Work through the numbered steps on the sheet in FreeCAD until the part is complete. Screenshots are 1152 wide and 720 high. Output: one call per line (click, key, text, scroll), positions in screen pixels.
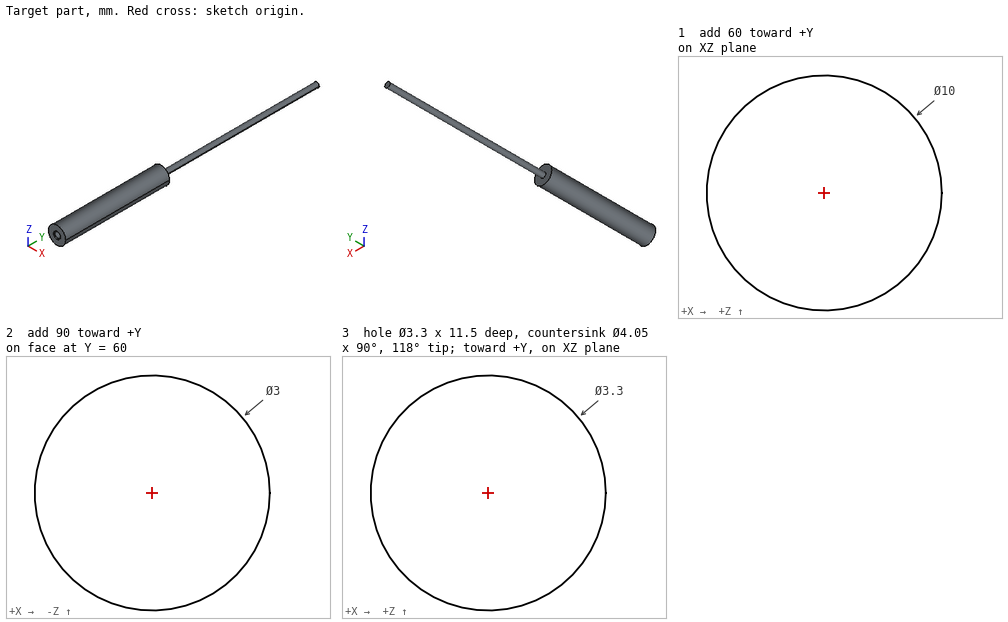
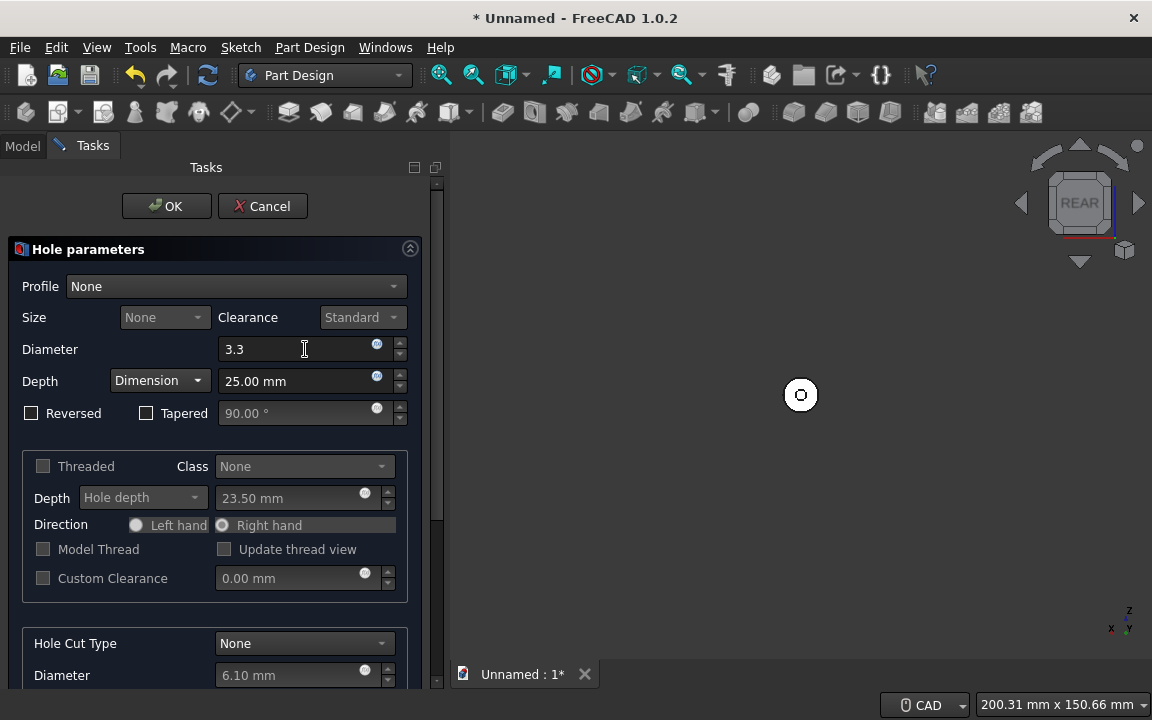
triple_click(305, 381)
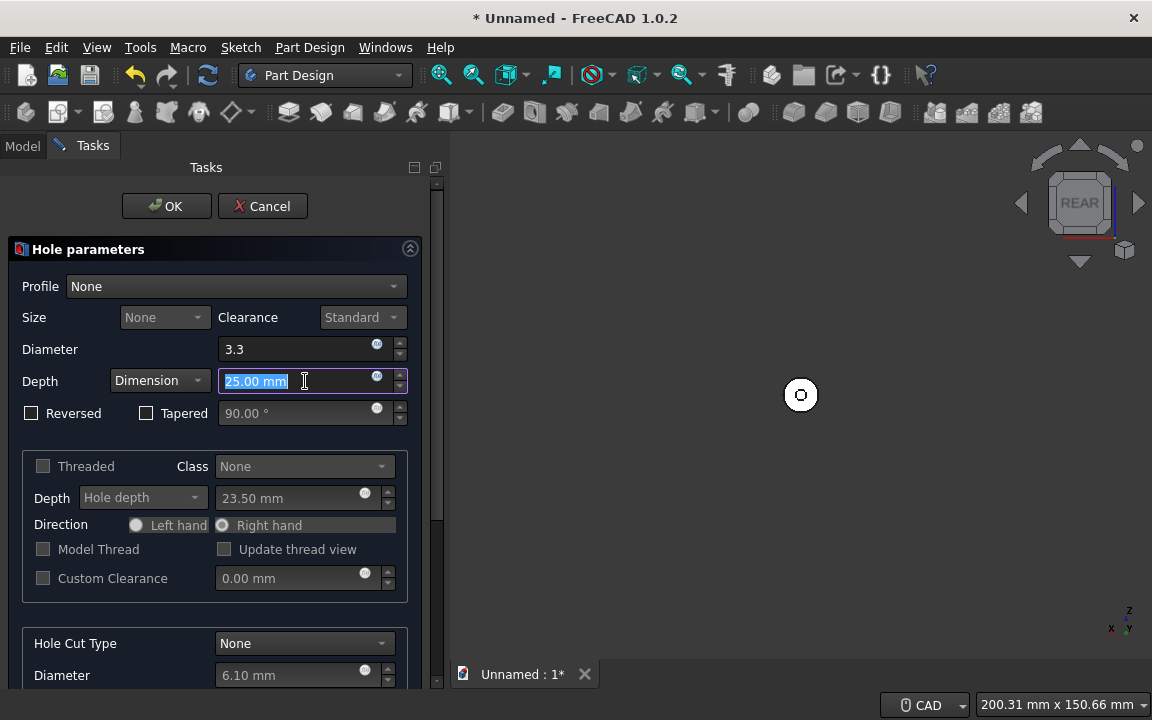
text(11.5)
key(Tab)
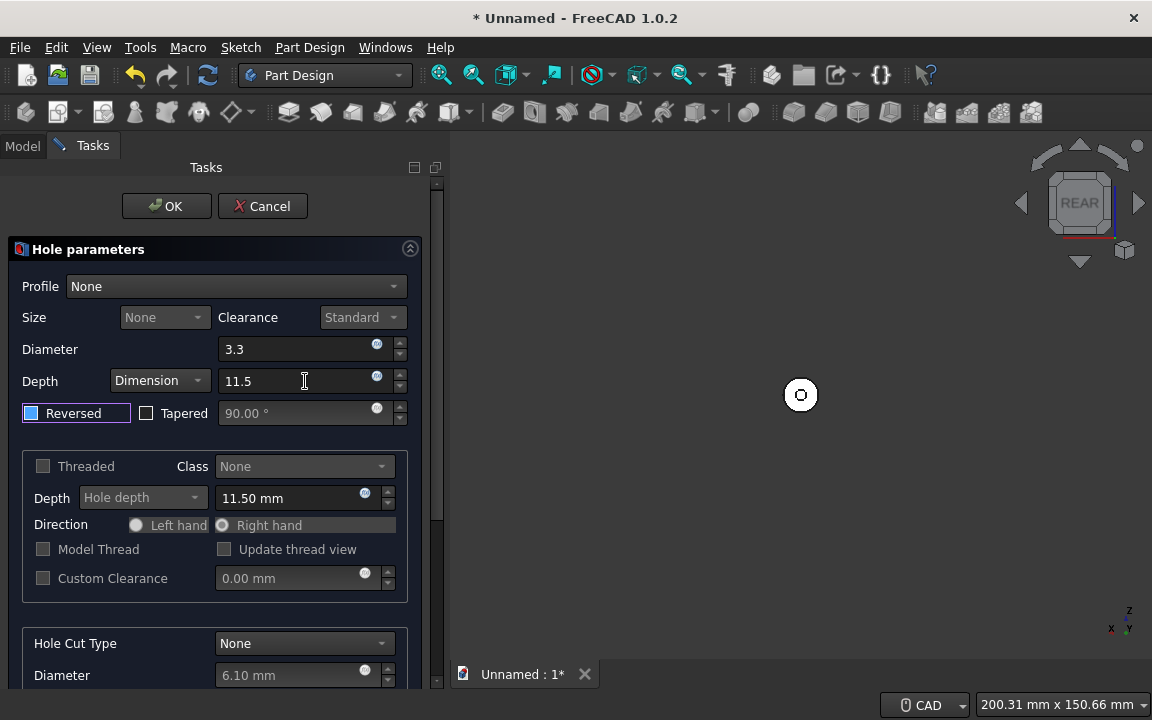
click(306, 644)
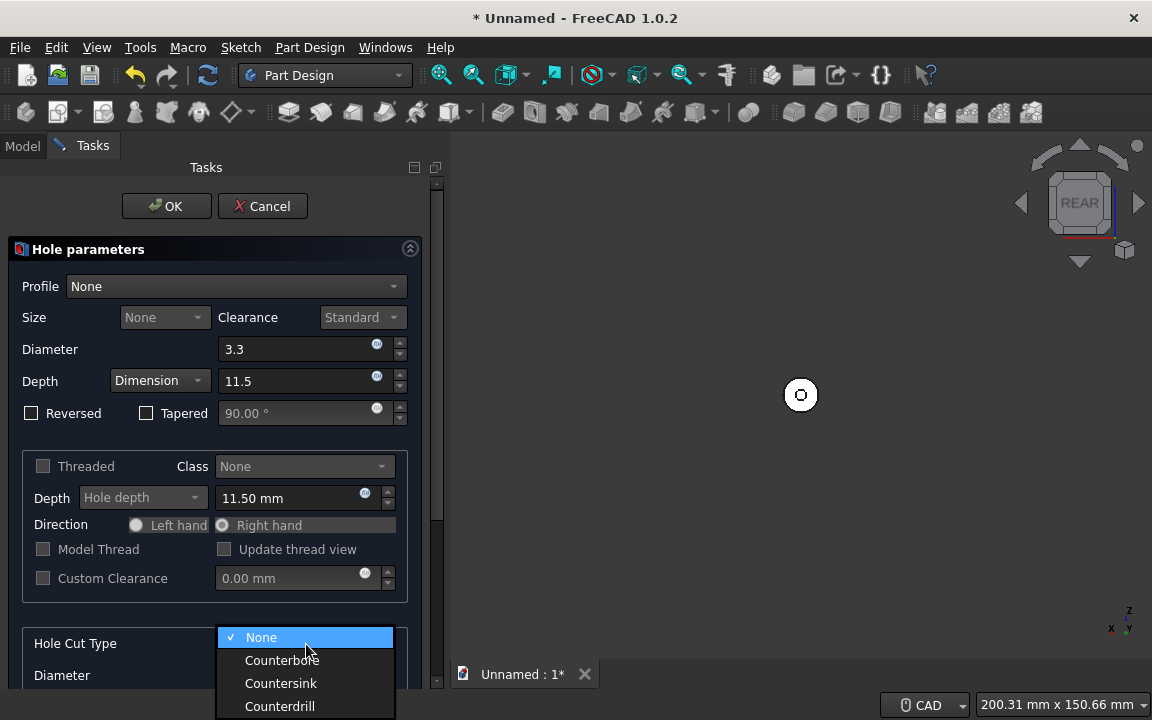
click(304, 684)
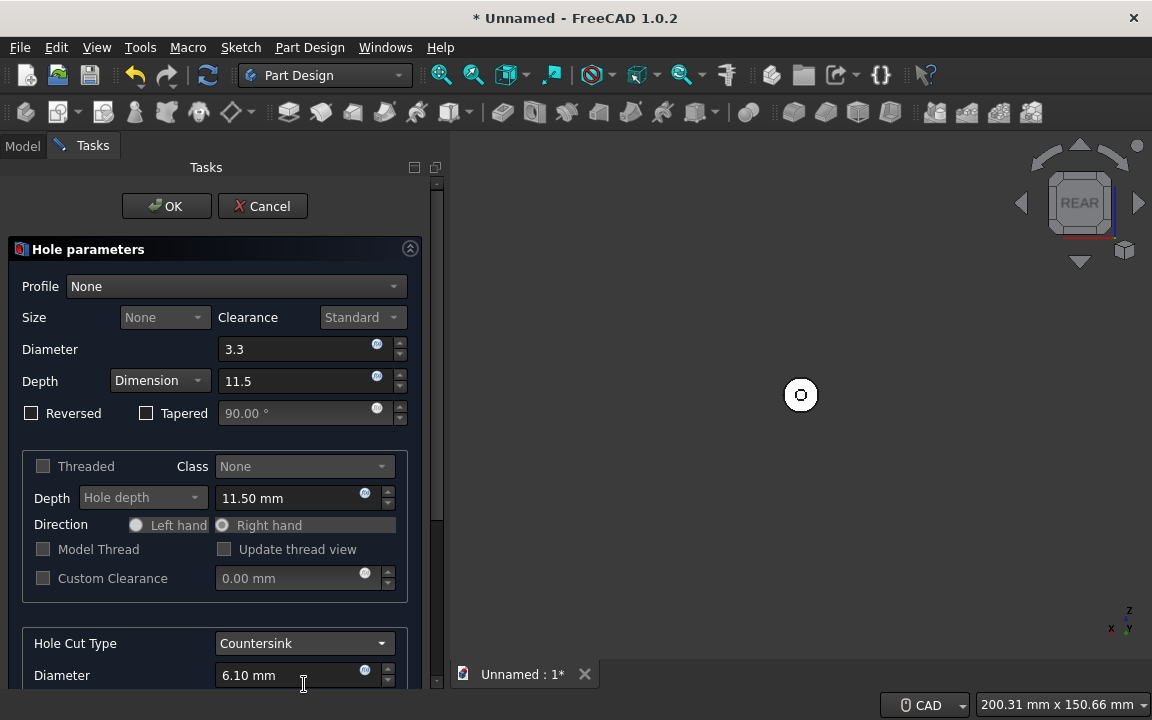
triple_click(298, 675)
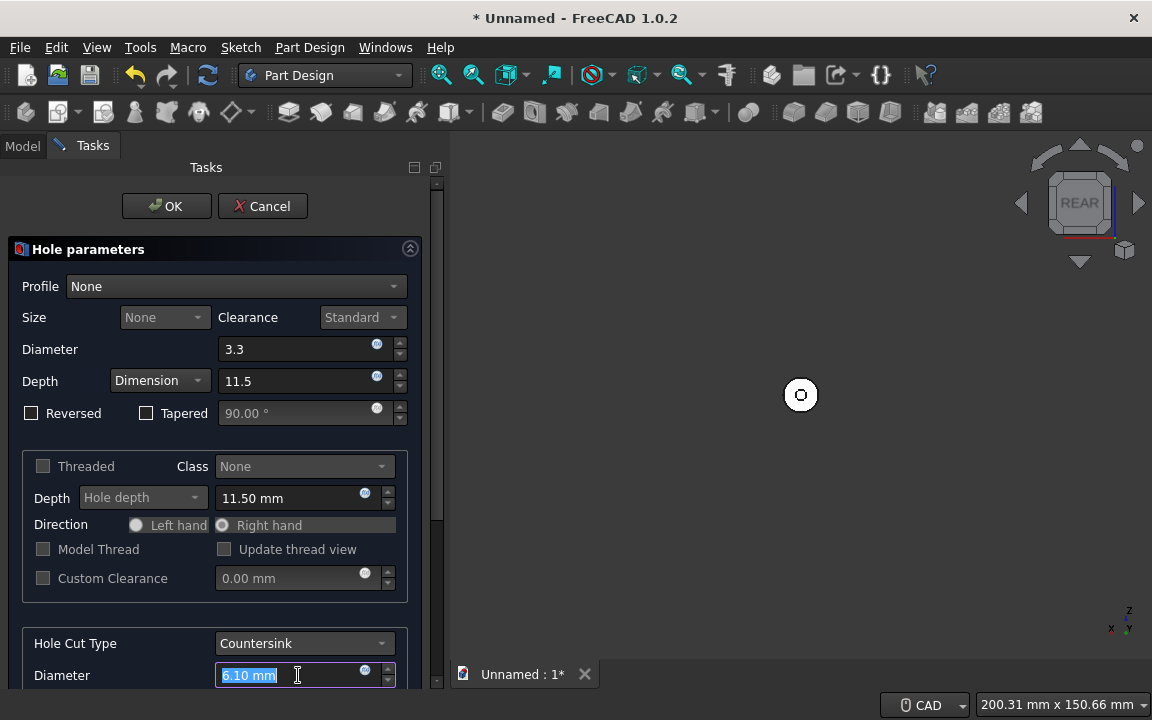
text(4.05)
key(Tab)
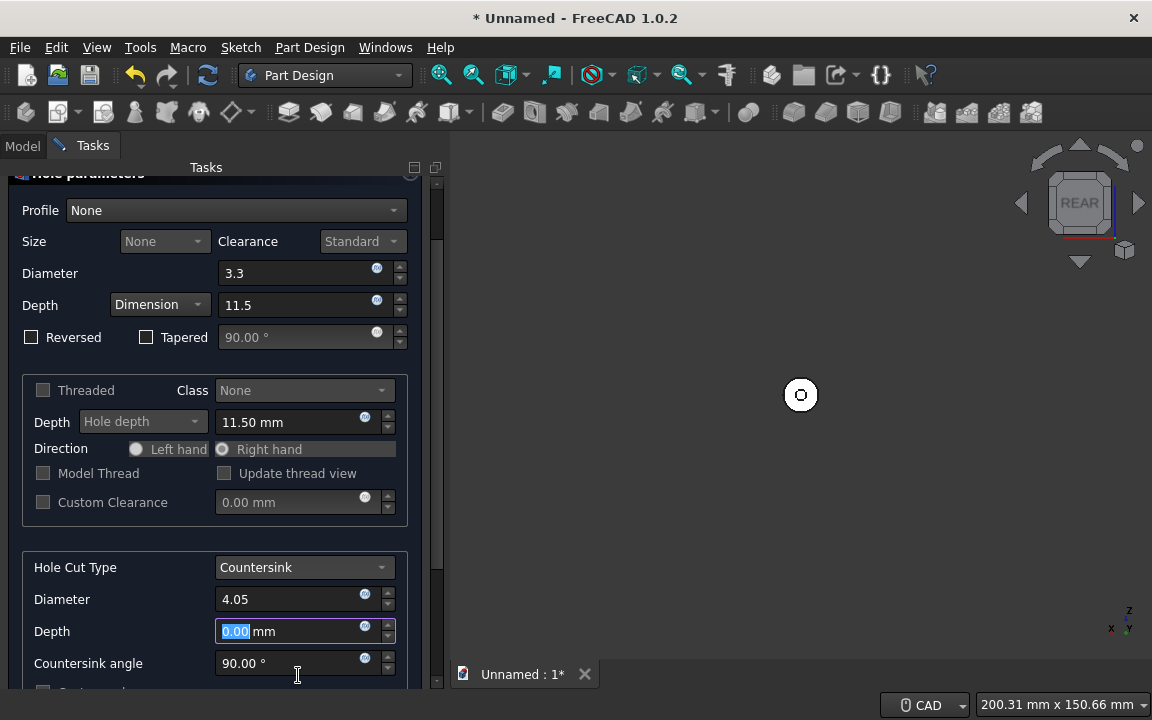
scroll(437, 432, up, 3)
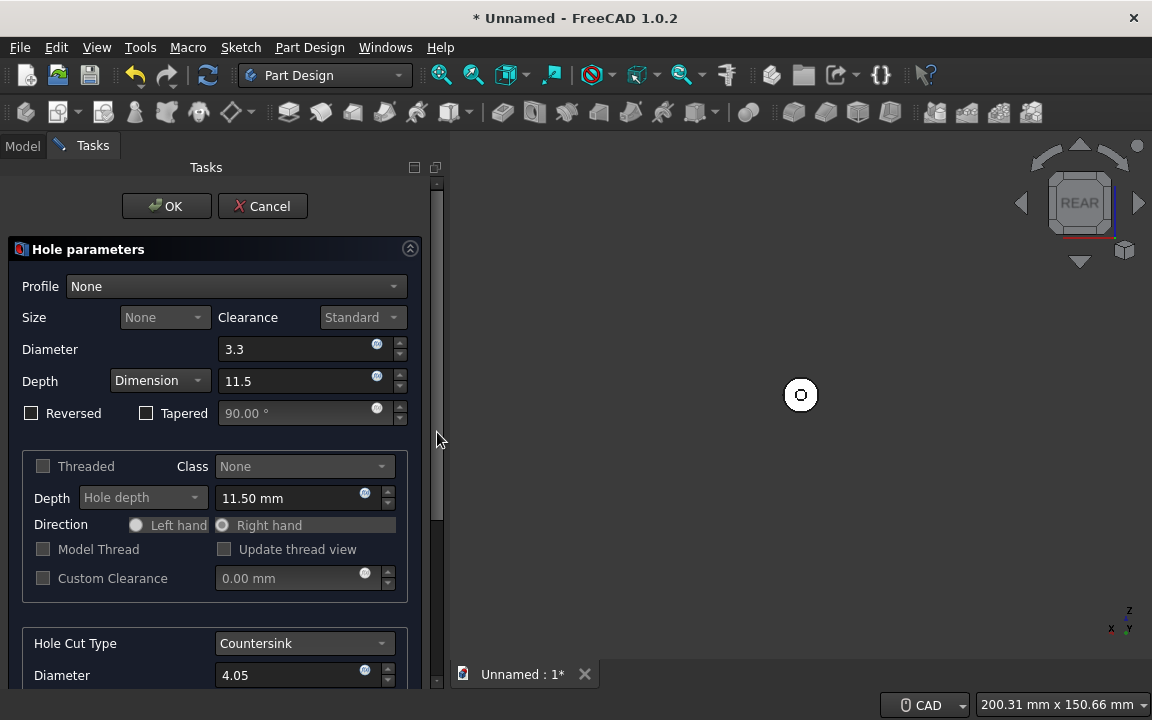
click(167, 206)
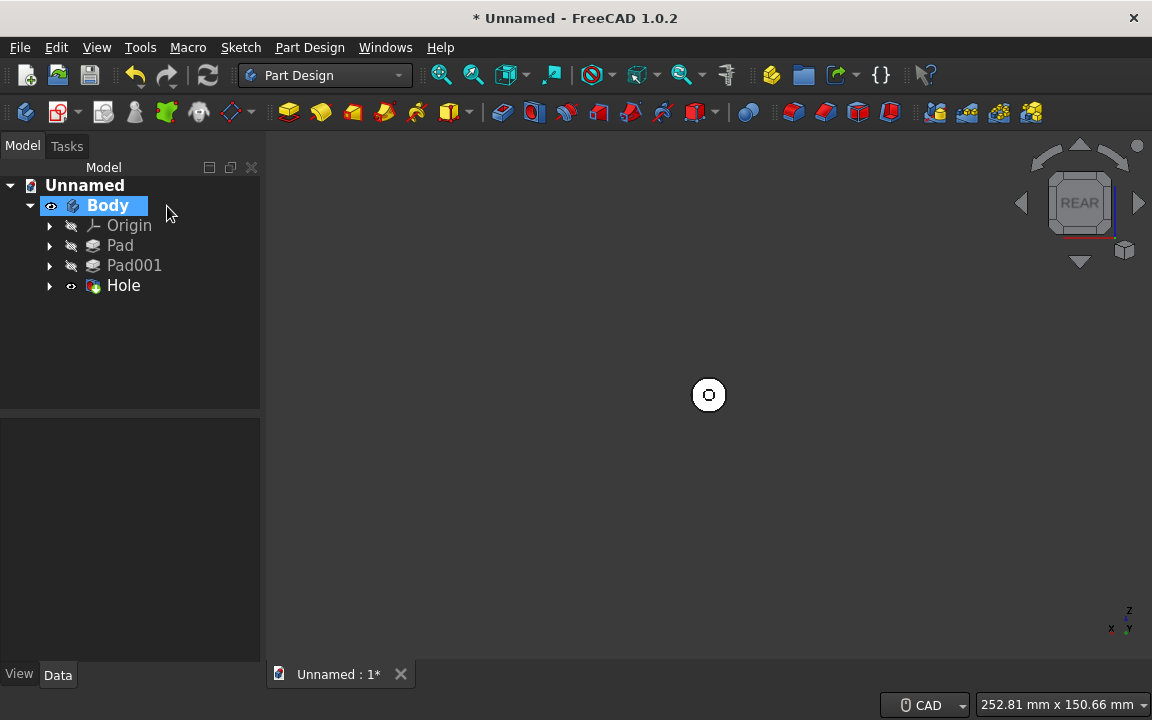
key(0)